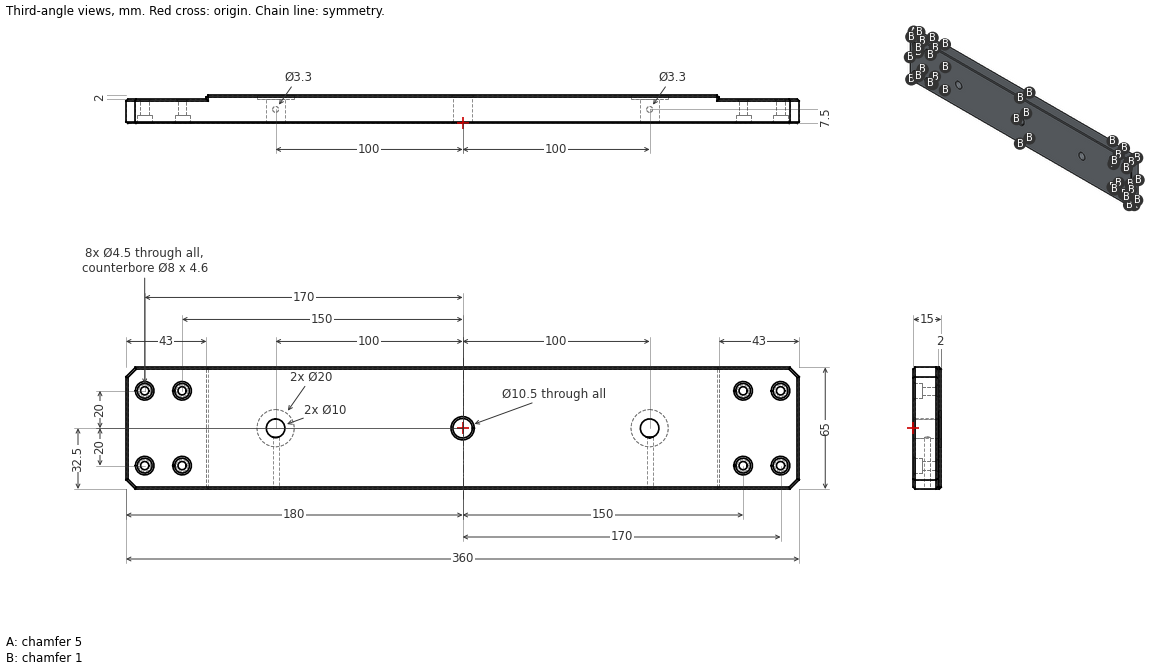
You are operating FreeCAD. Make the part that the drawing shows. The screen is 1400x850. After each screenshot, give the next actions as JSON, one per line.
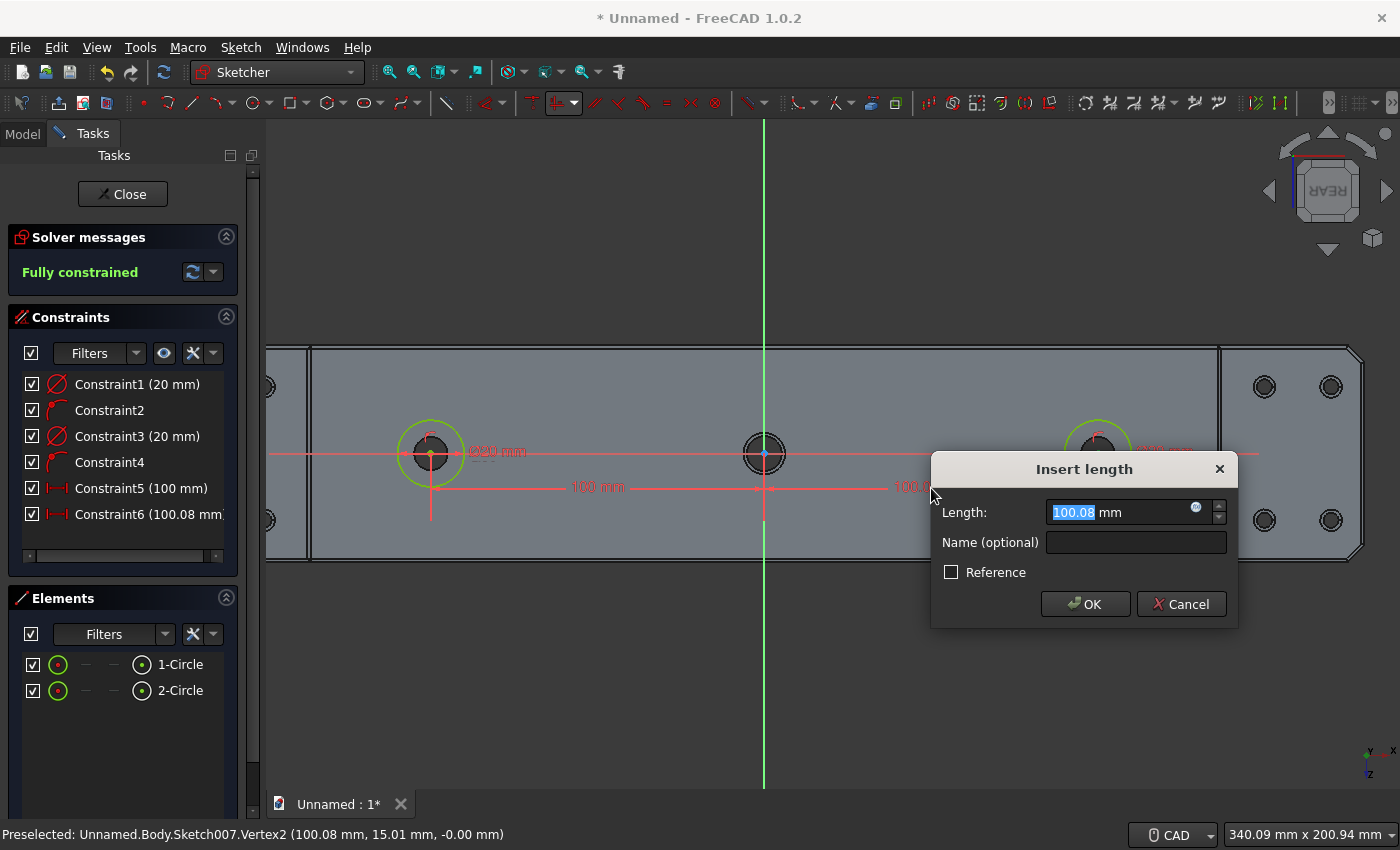
{"action": "type", "text": "100"}
{"action": "key", "text": "Return"}
{"action": "key", "text": "Escape"}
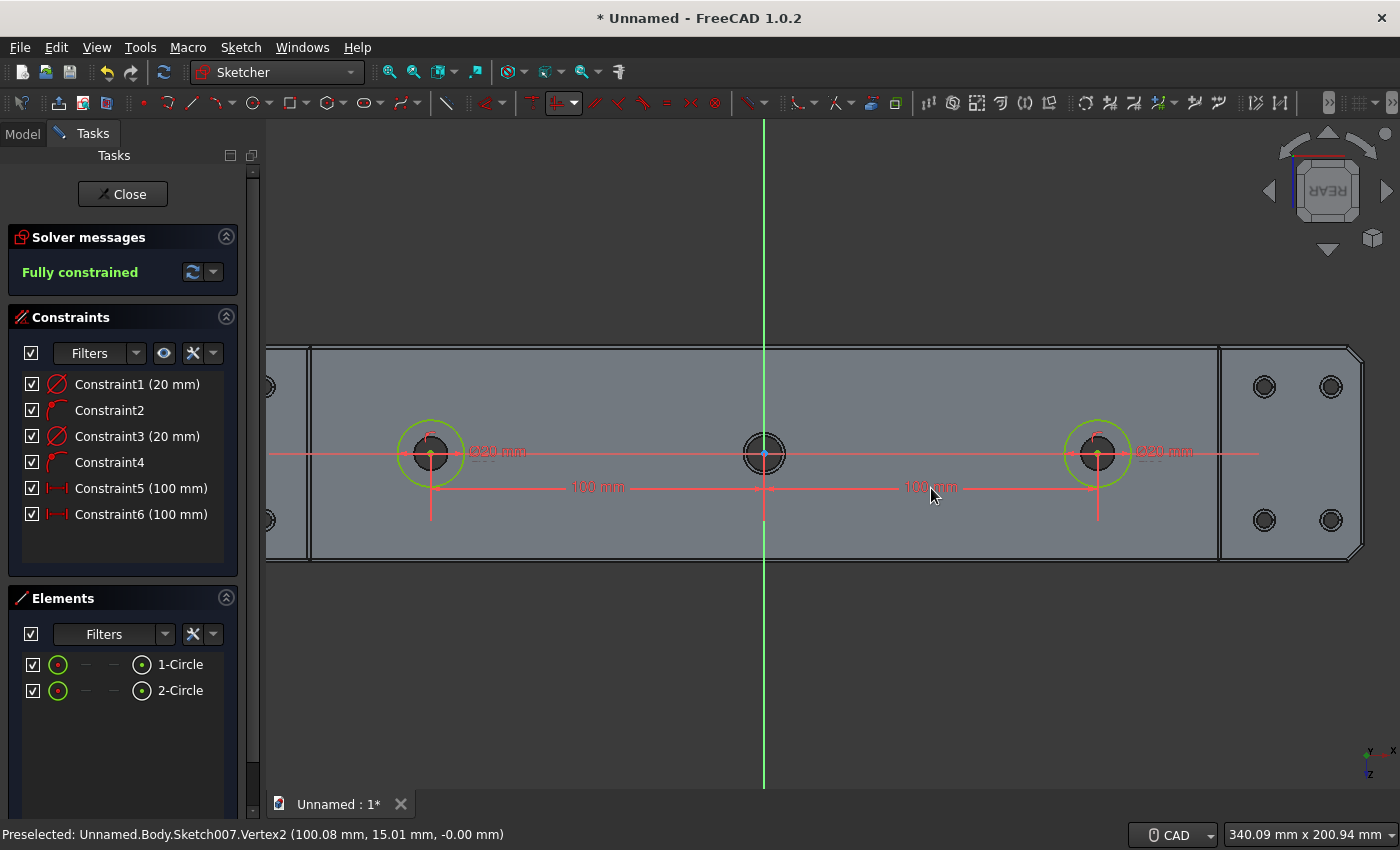
{"action": "left_click", "coordinate": [123, 194]}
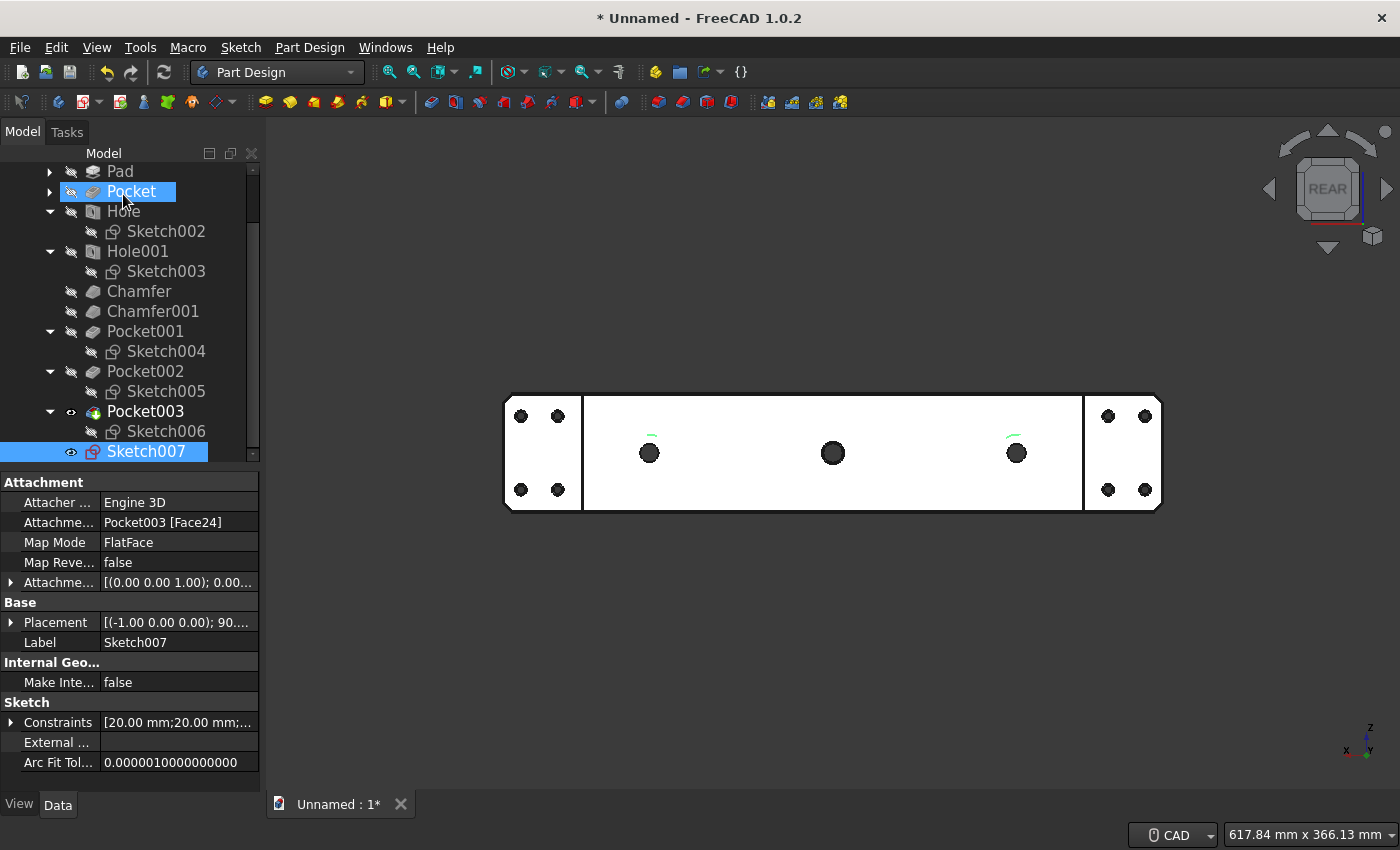
{"action": "left_click", "coordinate": [432, 102]}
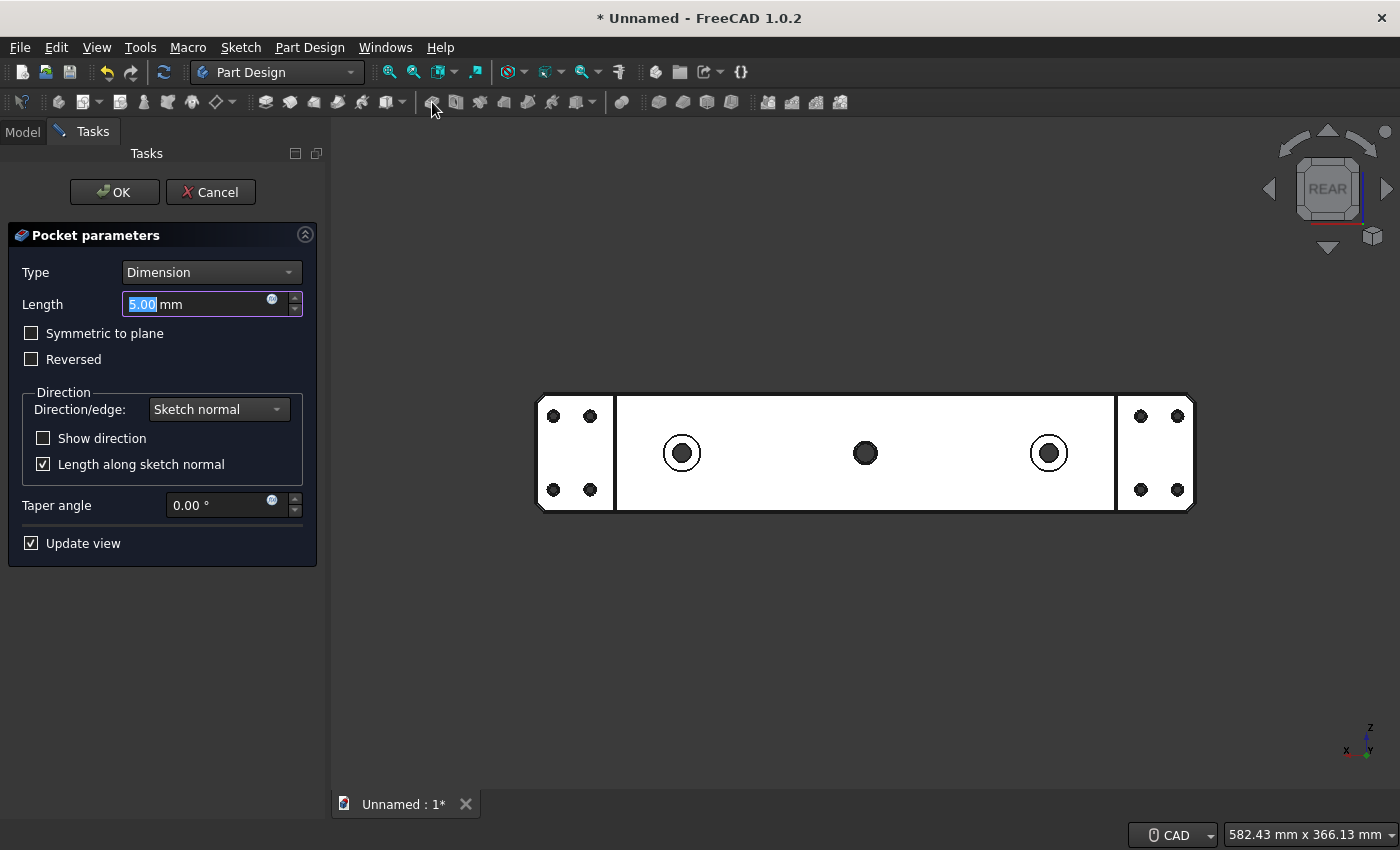
{"action": "type", "text": "2"}
{"action": "key", "text": "Tab"}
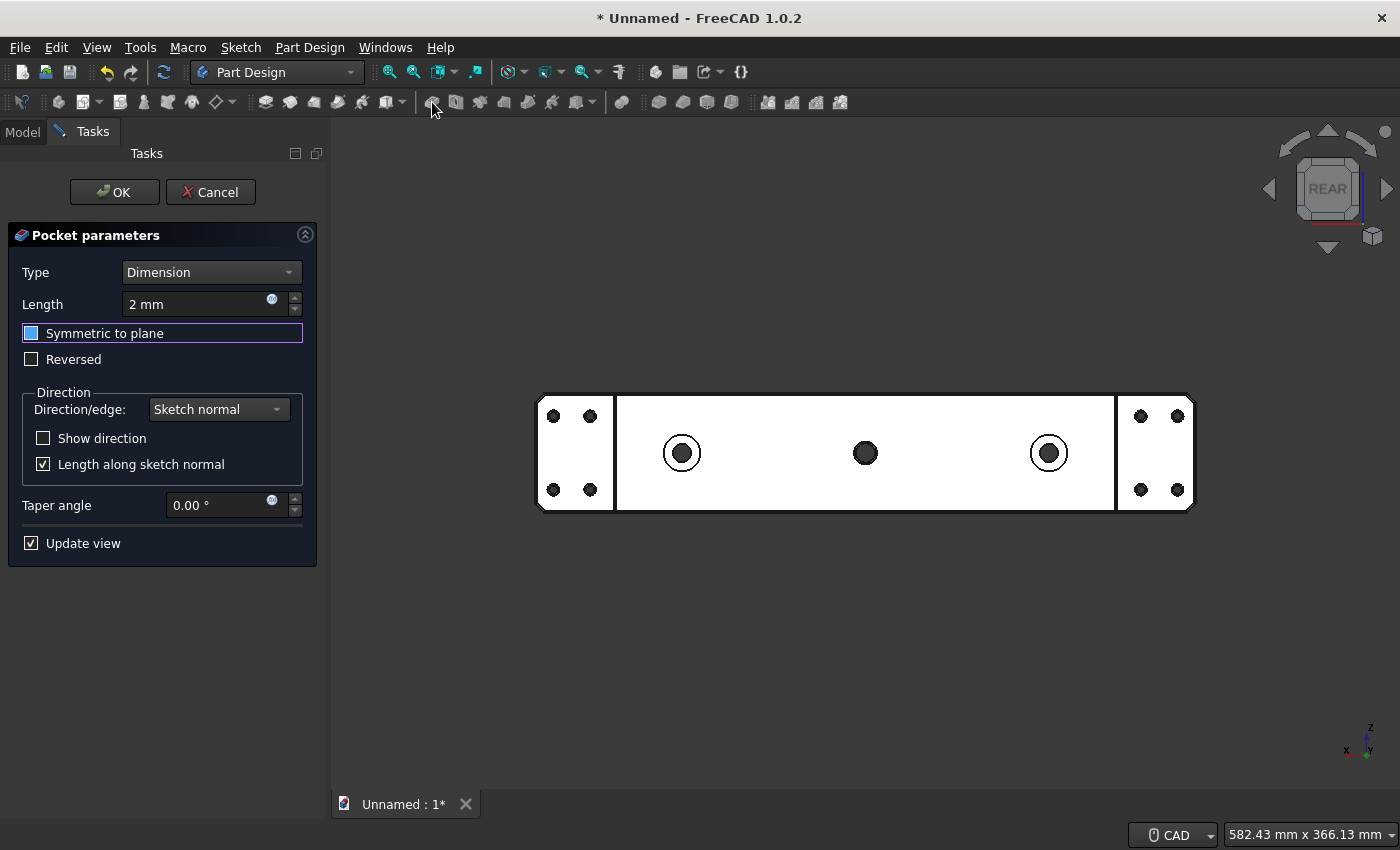
{"action": "left_click", "coordinate": [115, 192]}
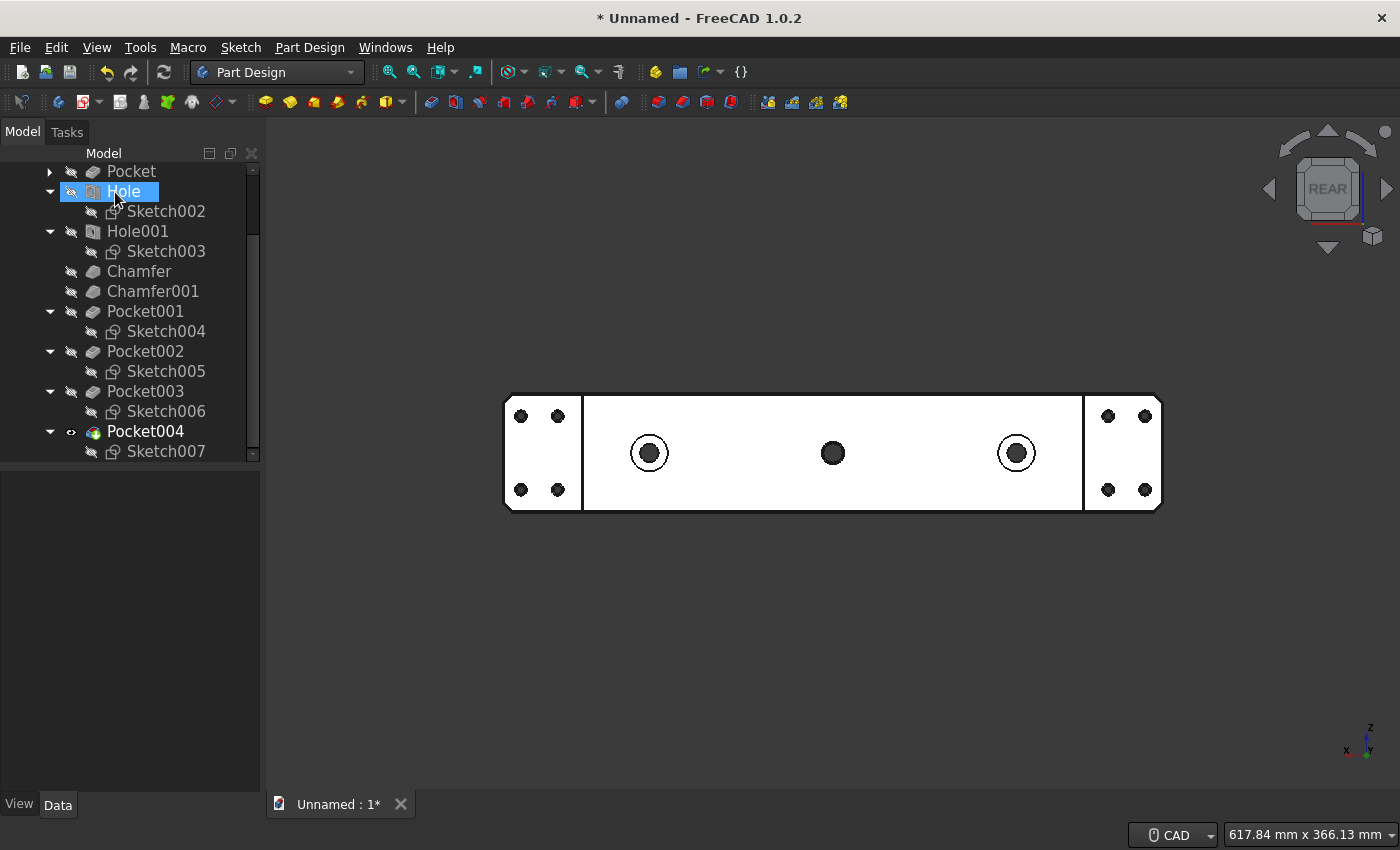
{"action": "key", "text": "0"}